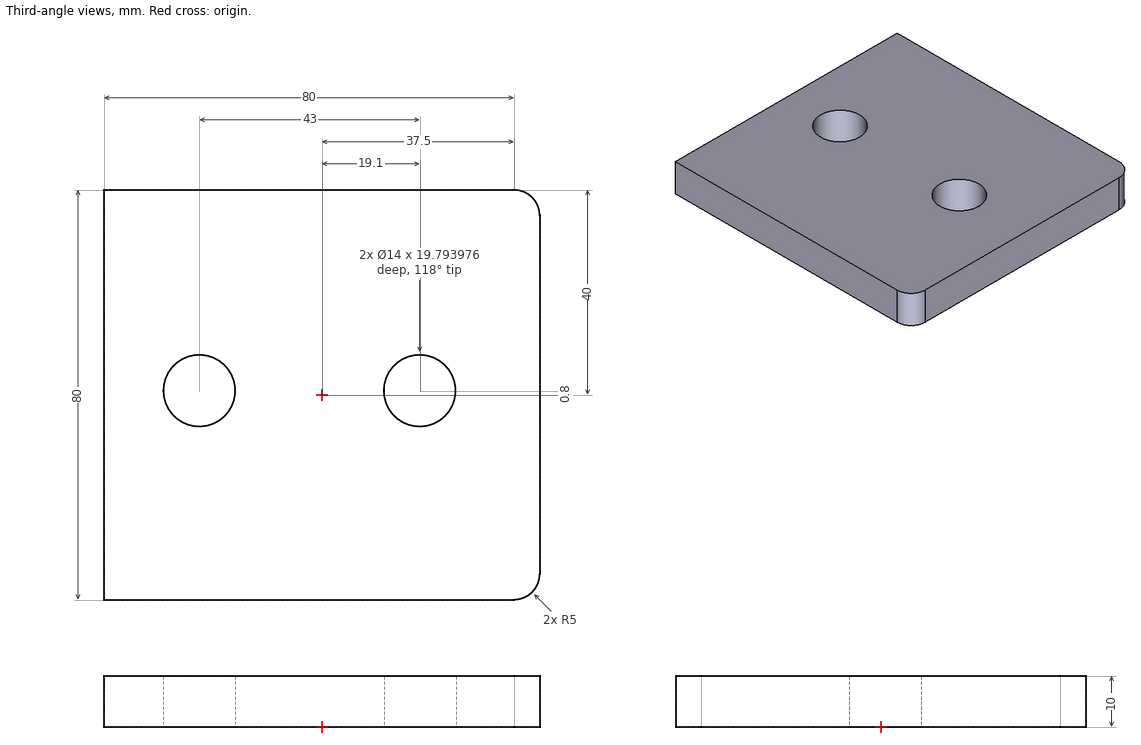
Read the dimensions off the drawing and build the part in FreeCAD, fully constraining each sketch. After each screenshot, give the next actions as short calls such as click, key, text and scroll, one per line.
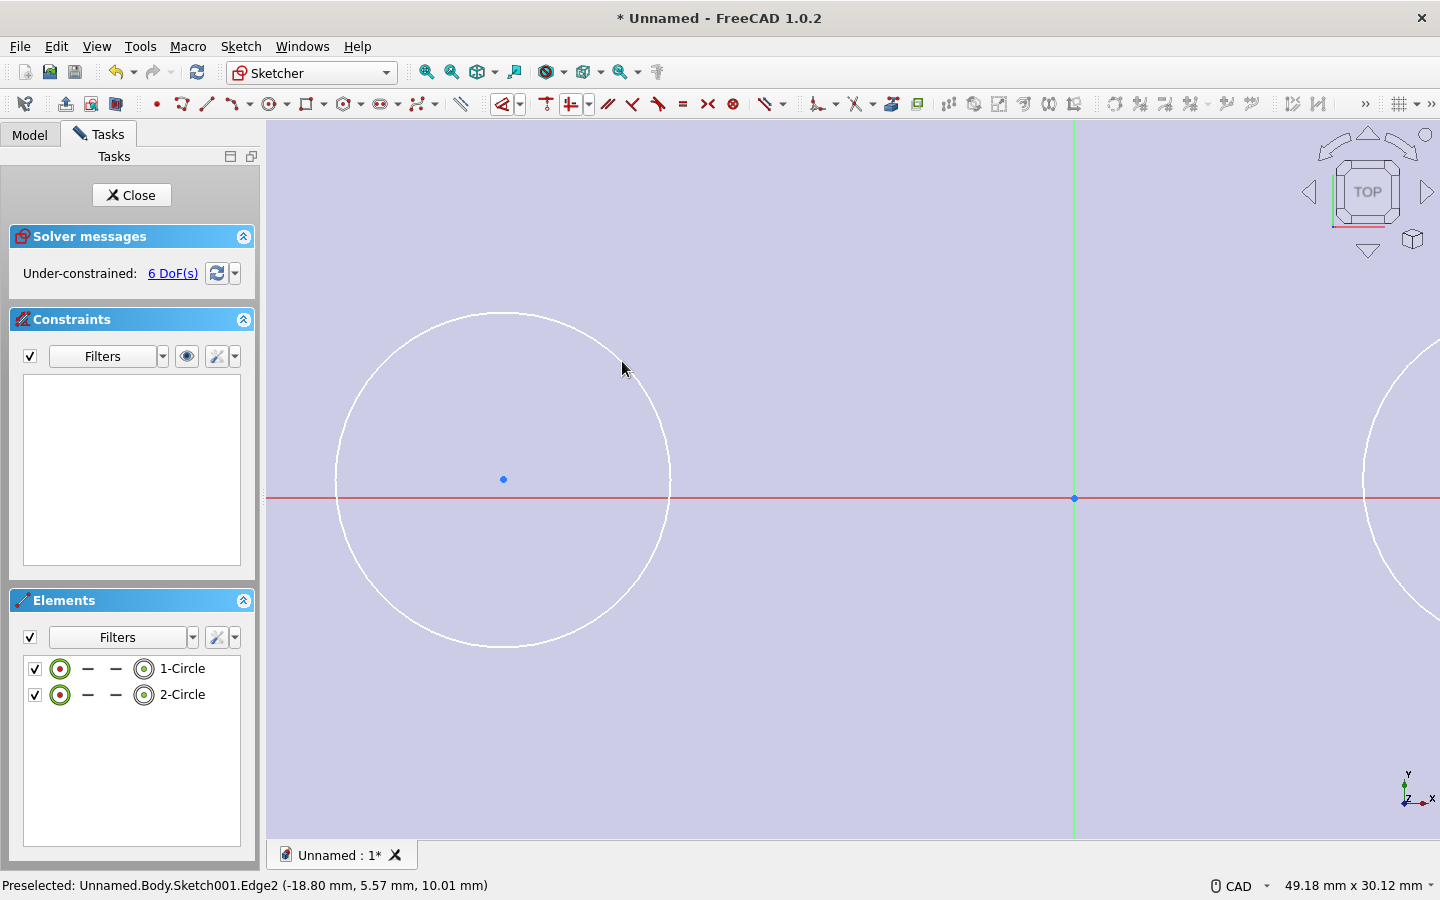
scroll(502, 480, down, 3)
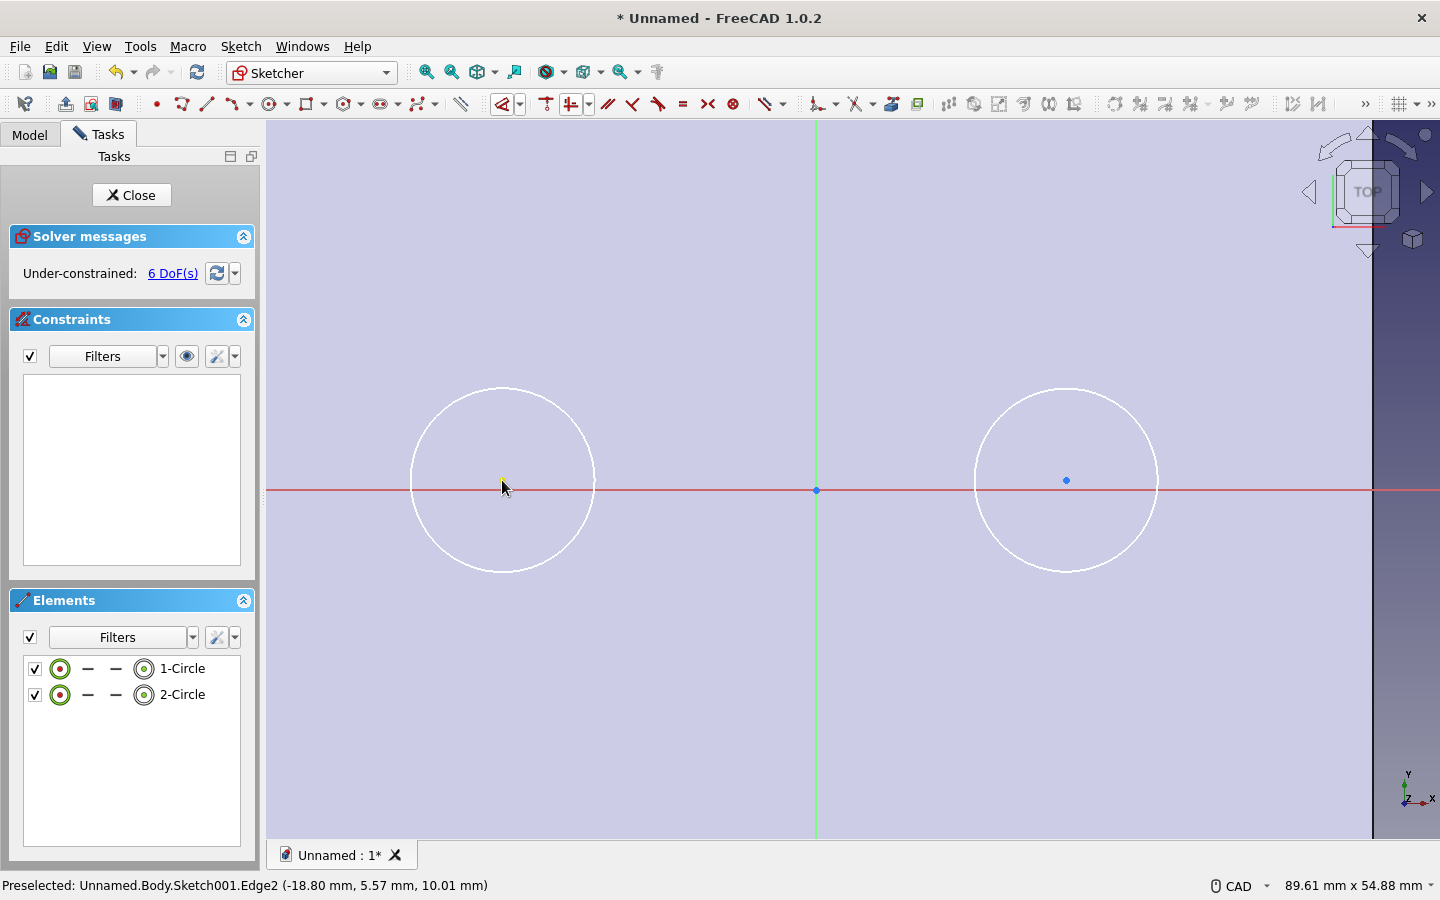
click(1131, 415)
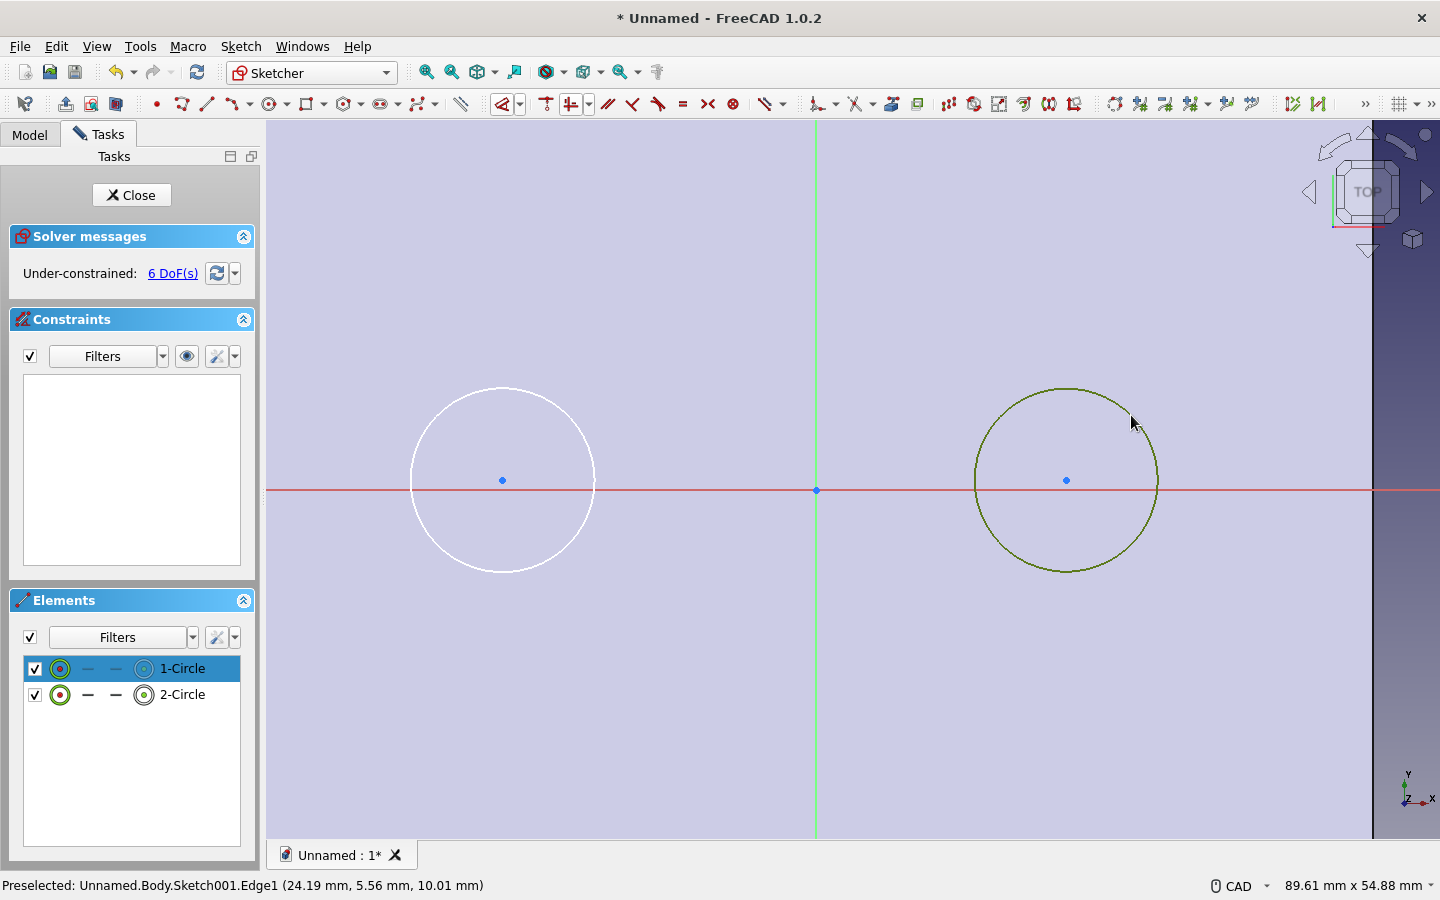
click(567, 415)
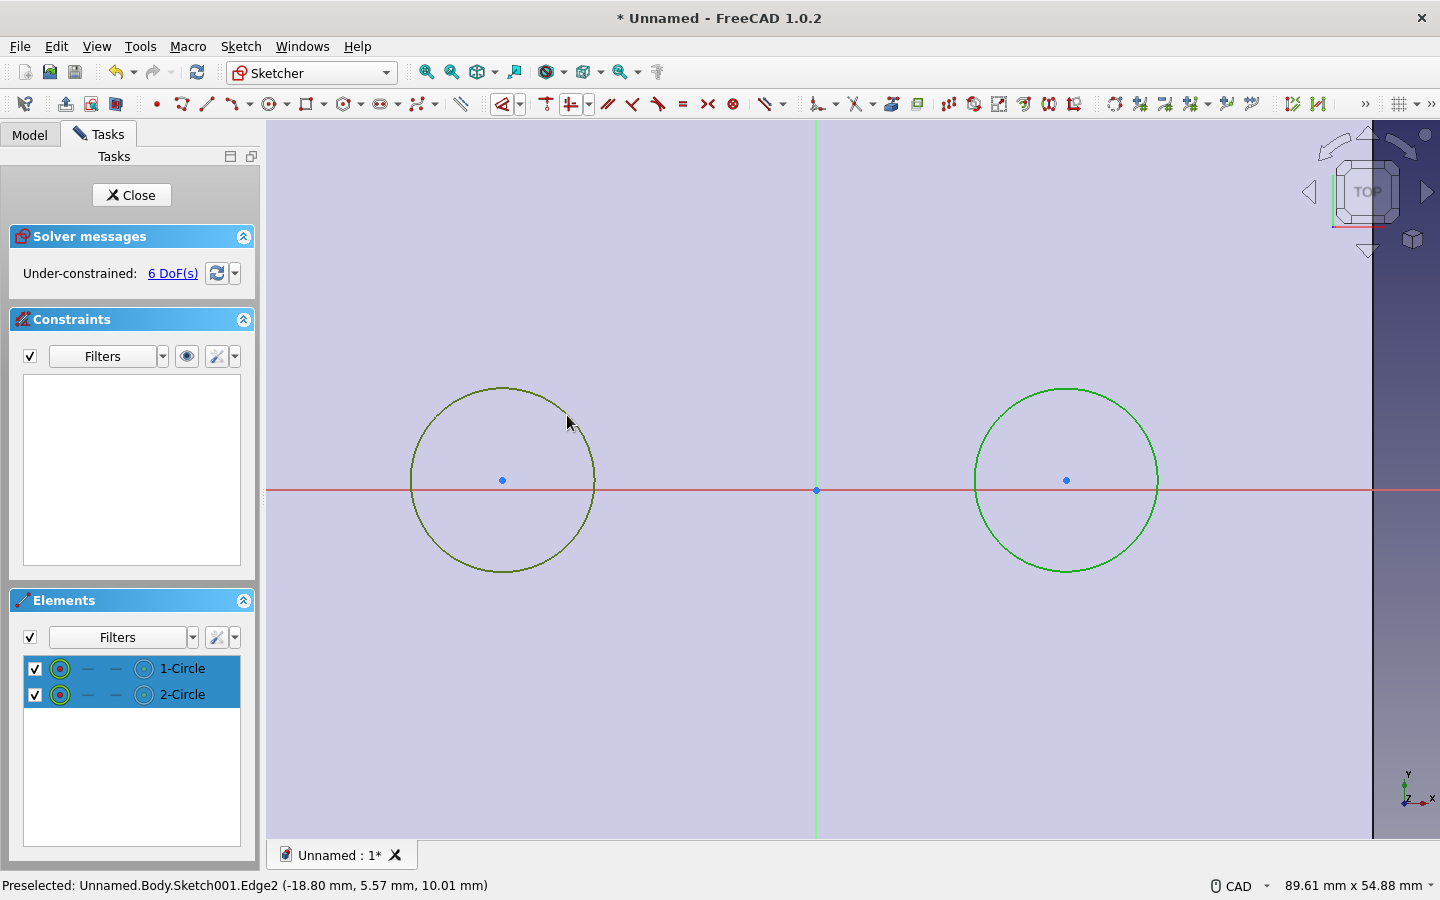
click(683, 104)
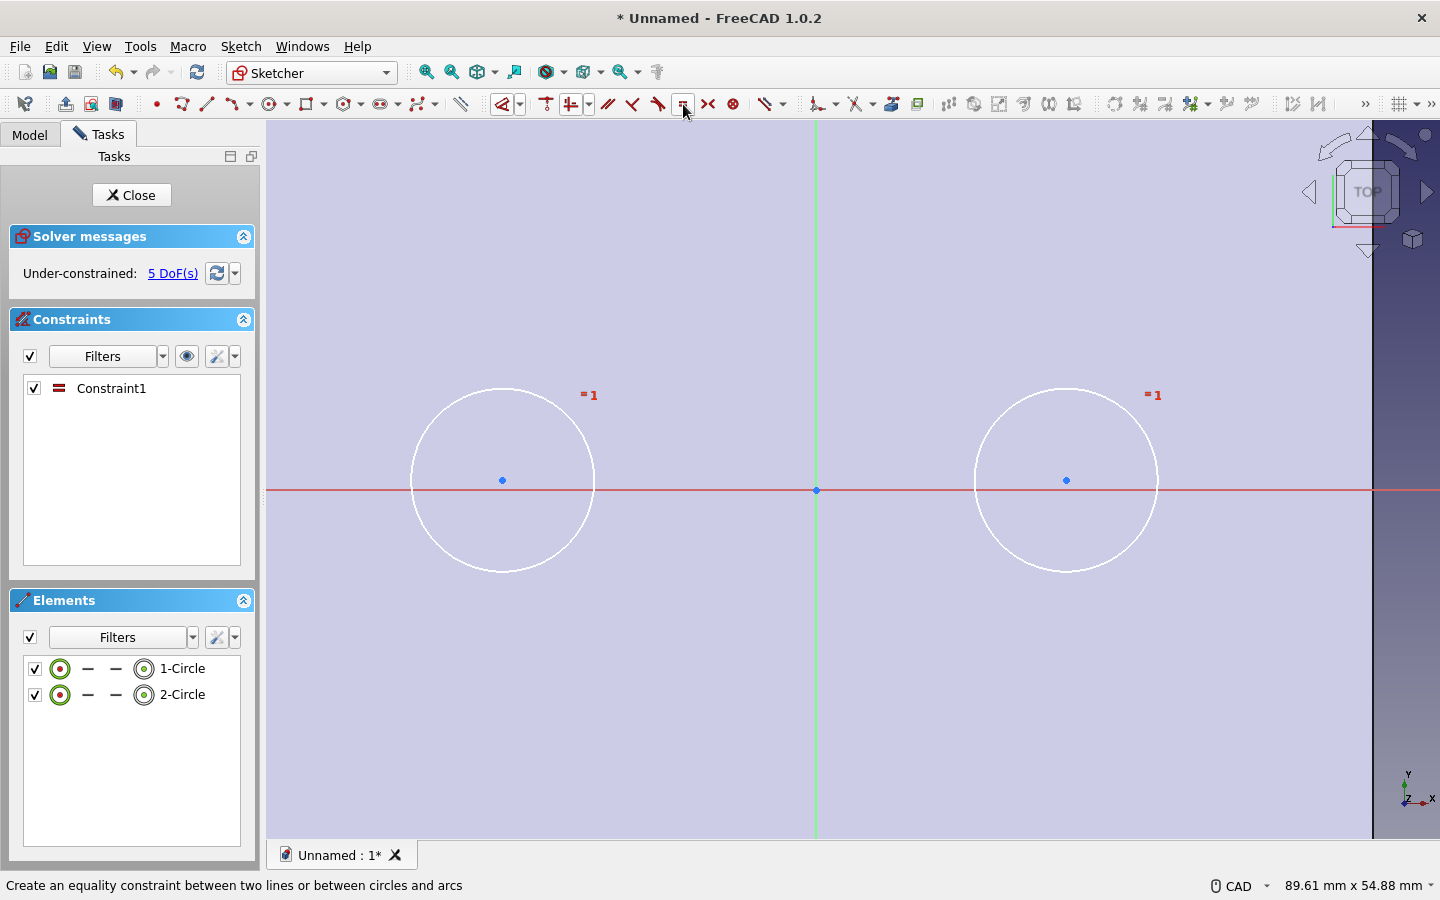
click(1131, 415)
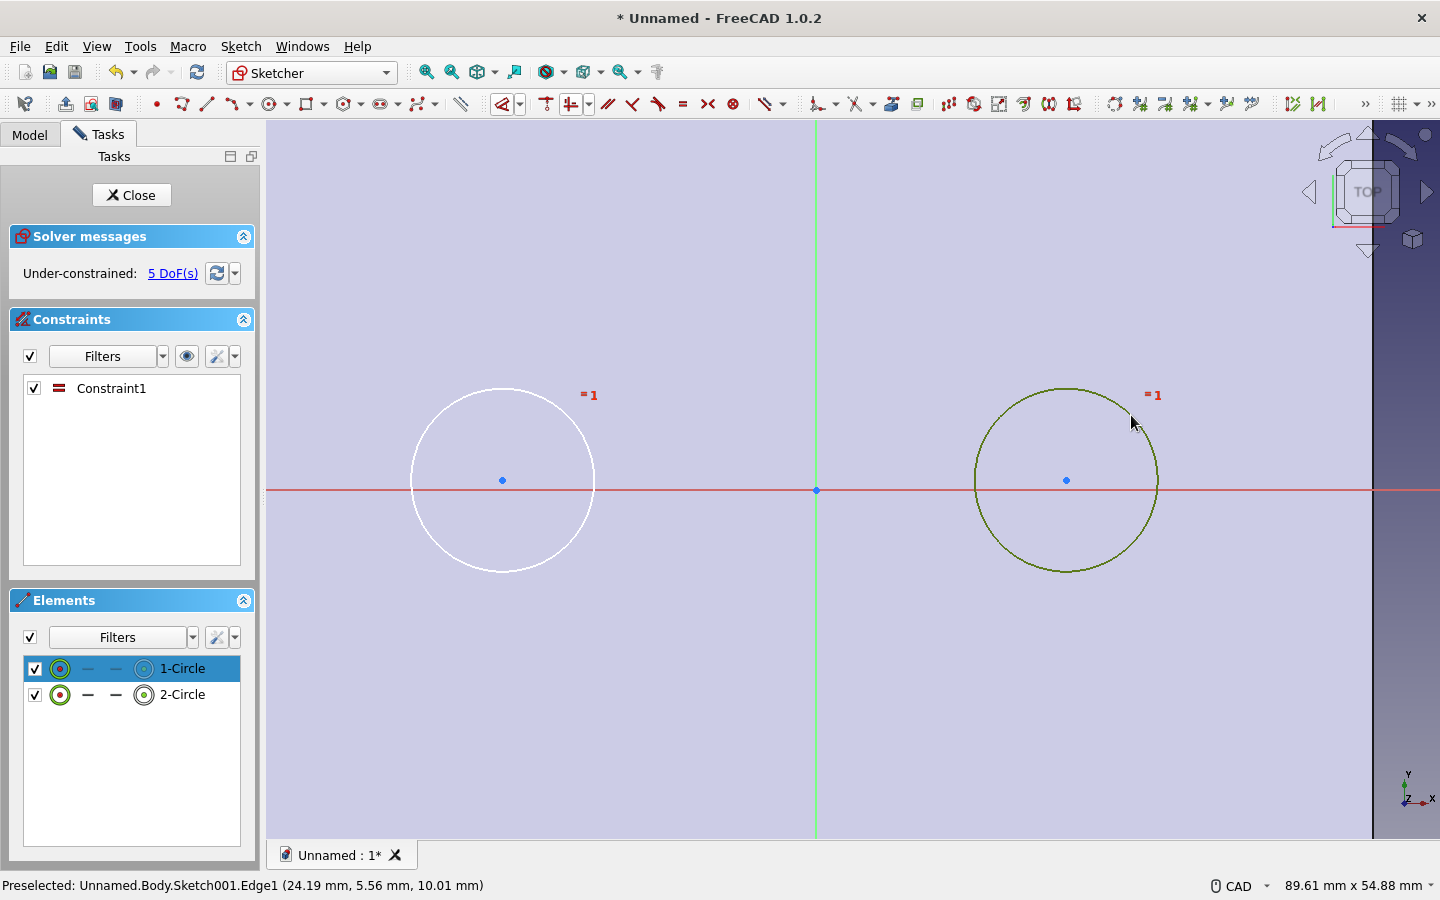
key(k)
key(o)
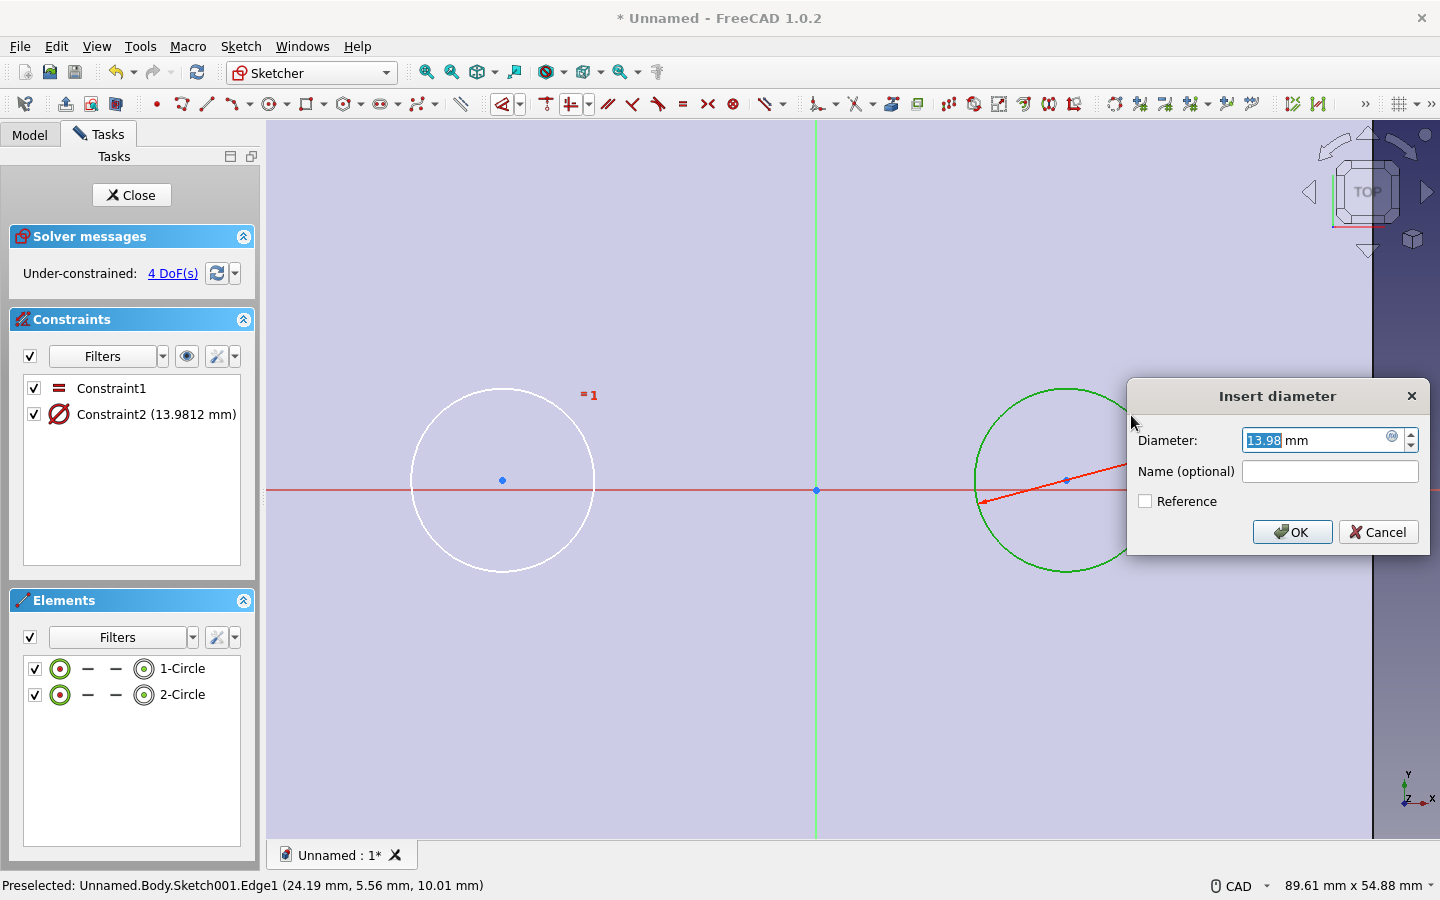
text(14)
key(Return)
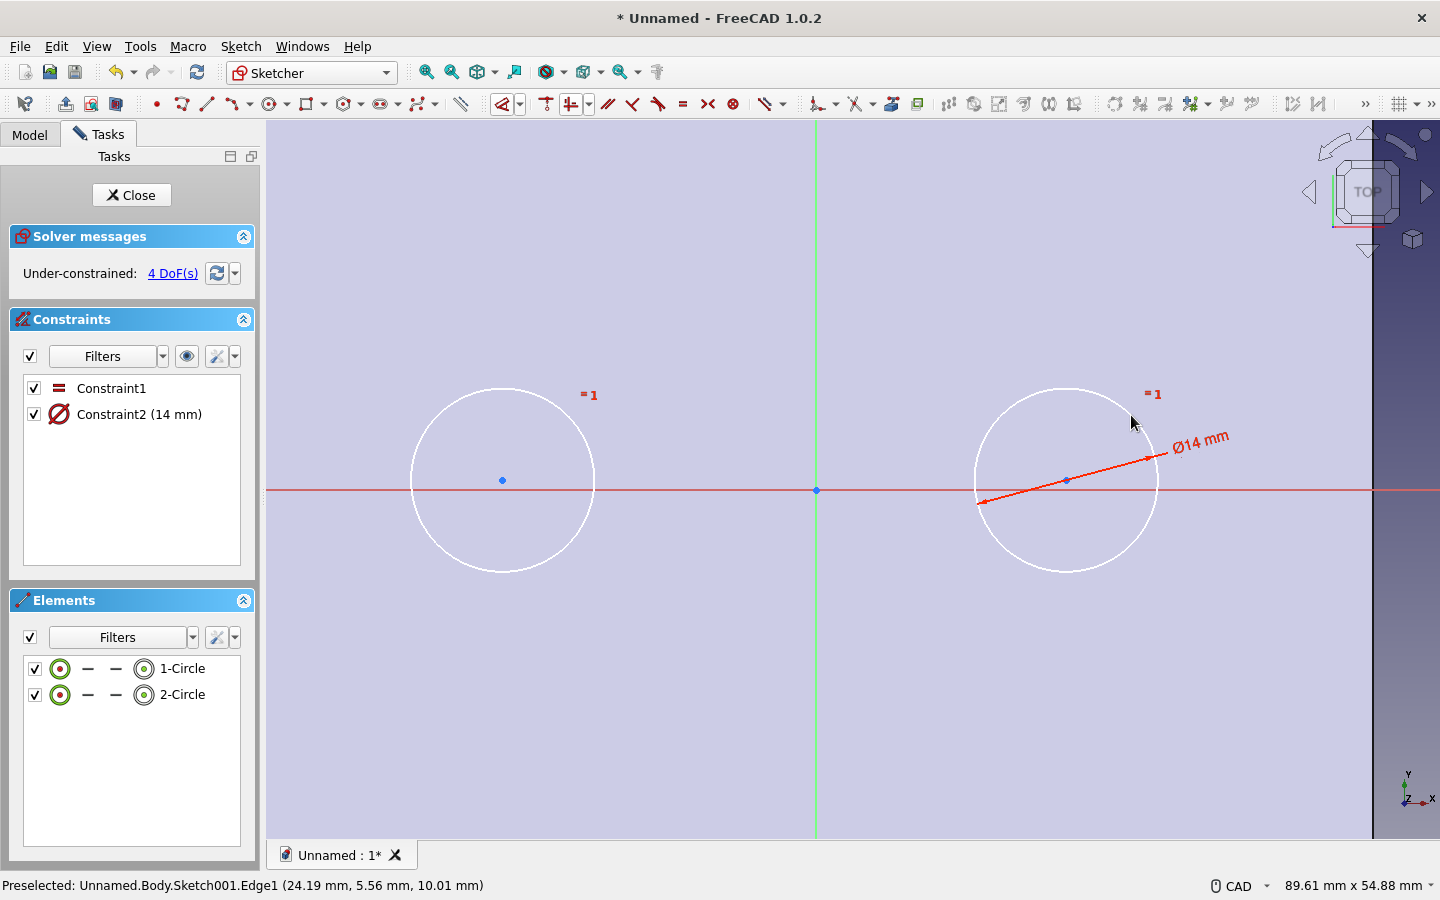
scroll(1066, 480, up, 7)